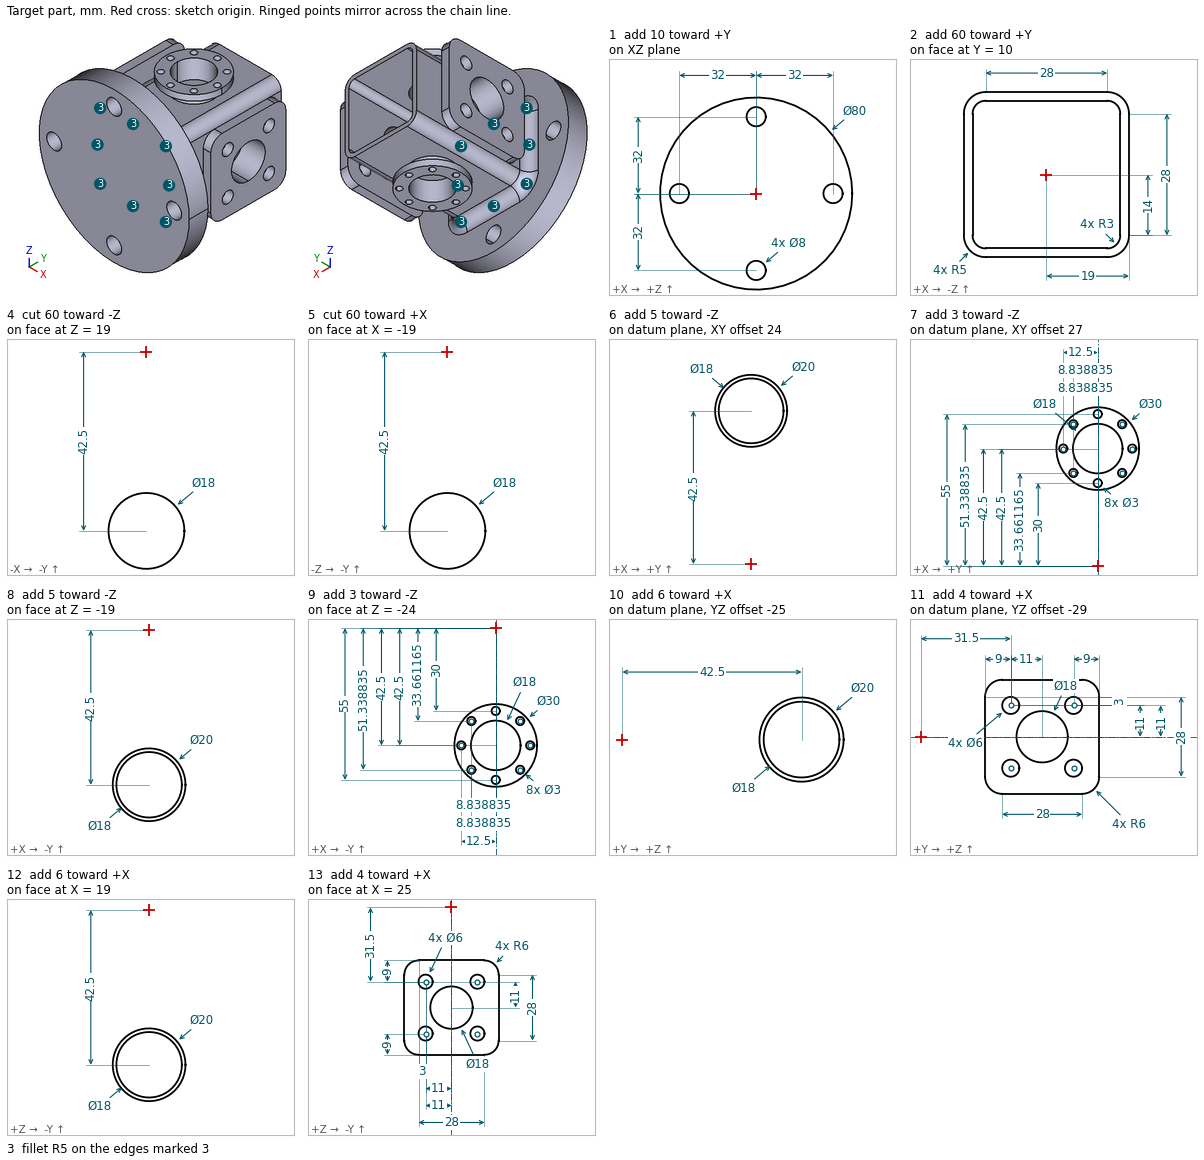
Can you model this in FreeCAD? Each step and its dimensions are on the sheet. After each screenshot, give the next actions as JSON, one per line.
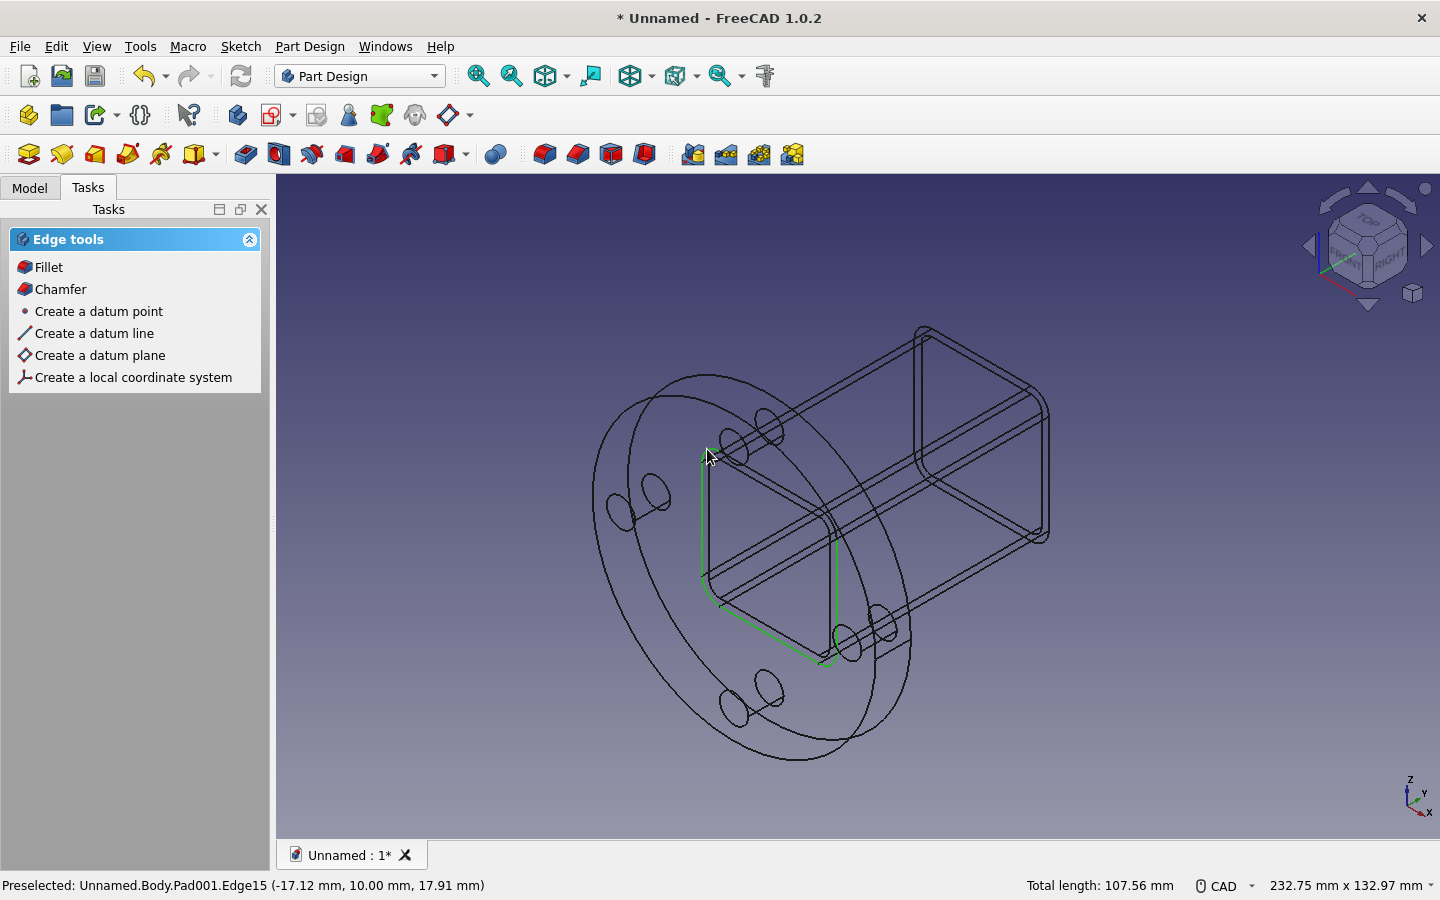
{"action": "left_click", "coordinate": [769, 479], "text": "ctrl"}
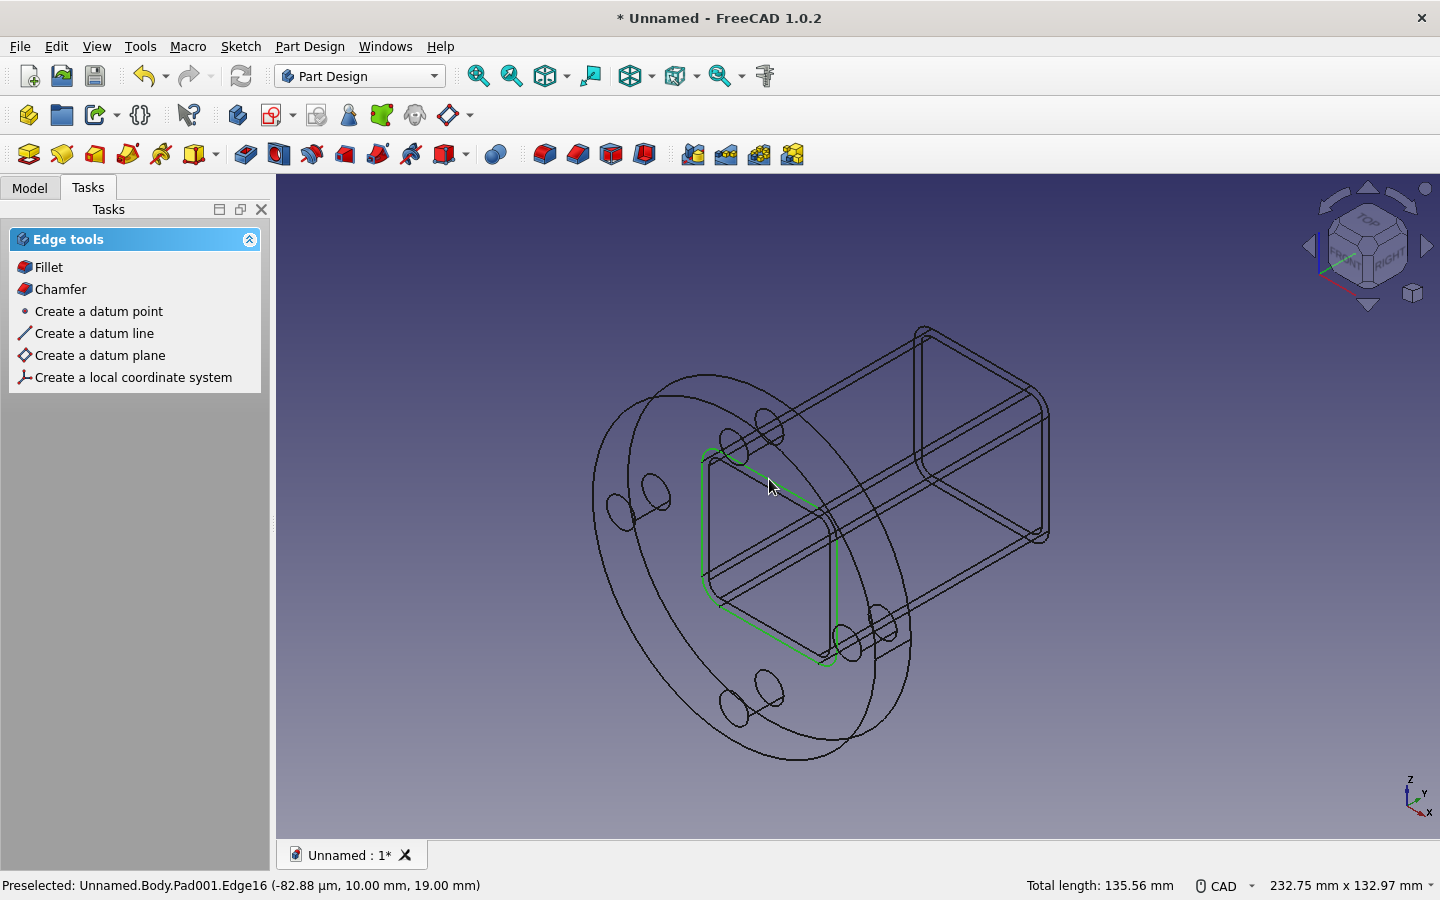
{"action": "key", "text": "2"}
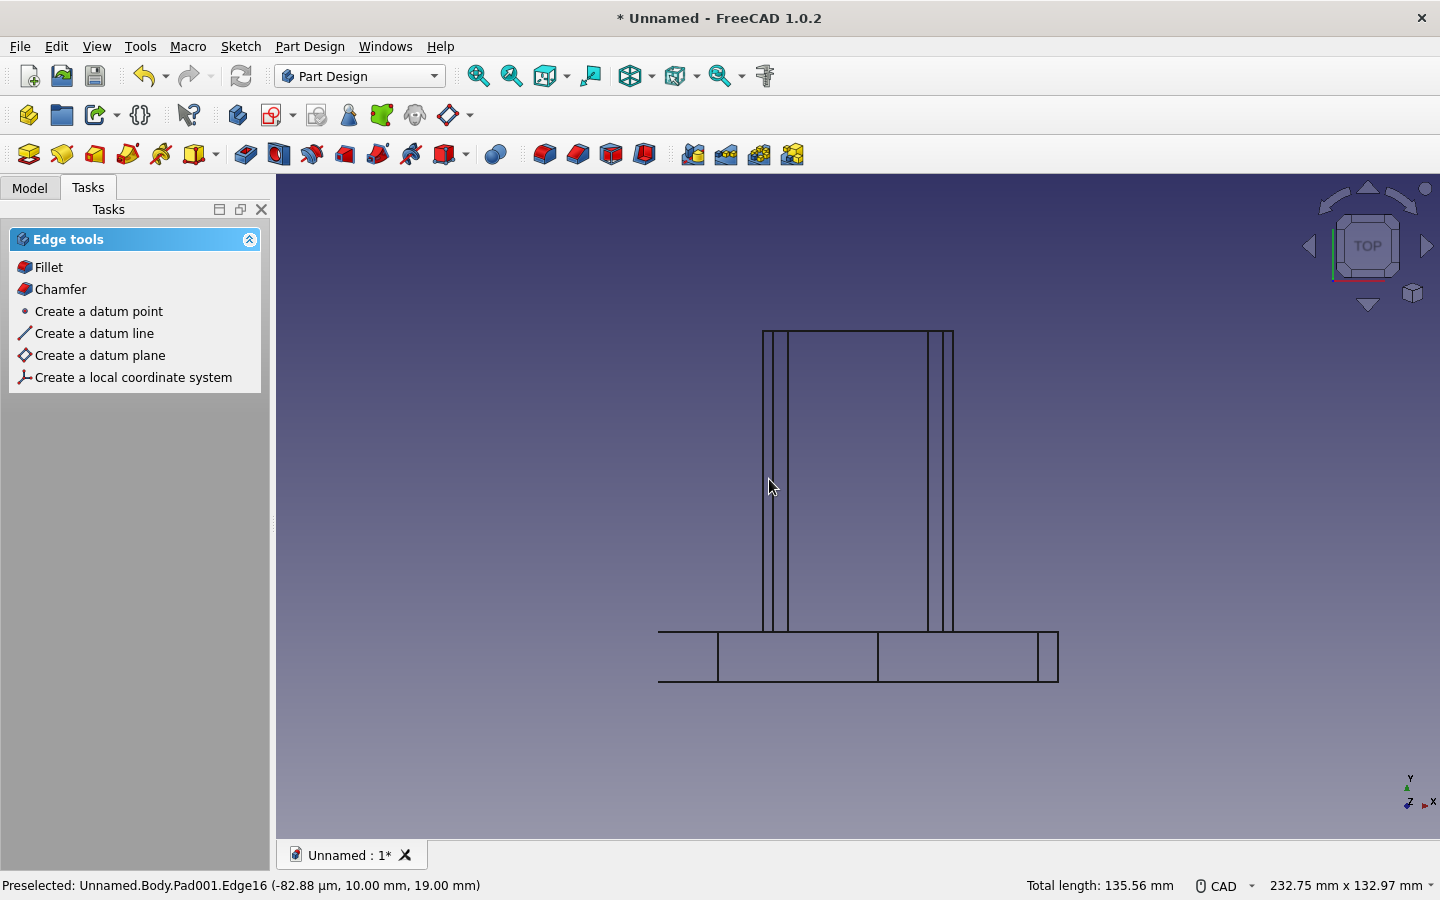
{"action": "key", "text": "1"}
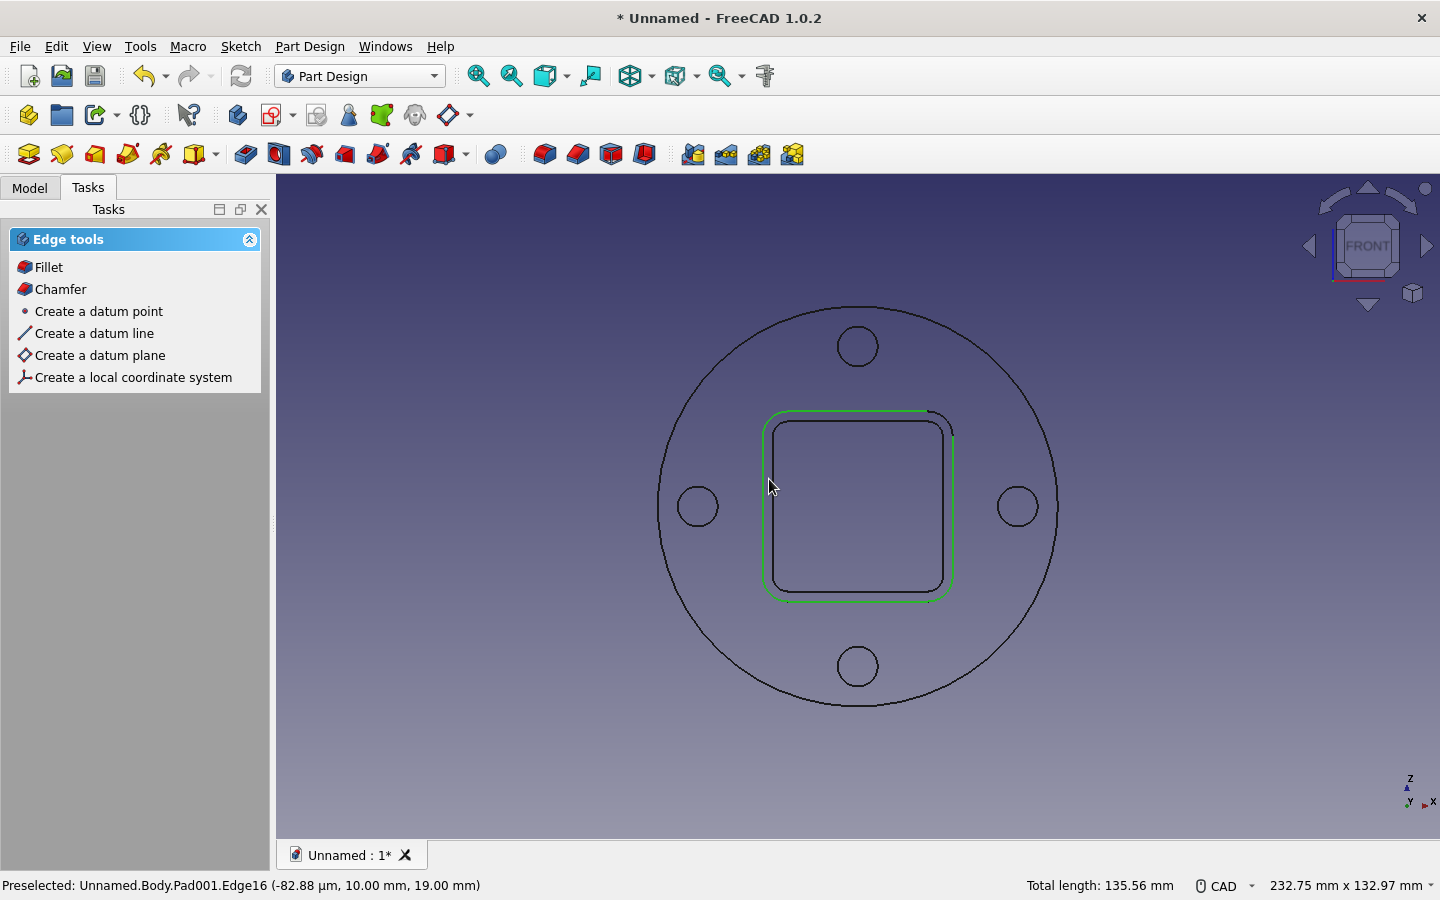
{"action": "left_click", "coordinate": [946, 418], "text": "ctrl"}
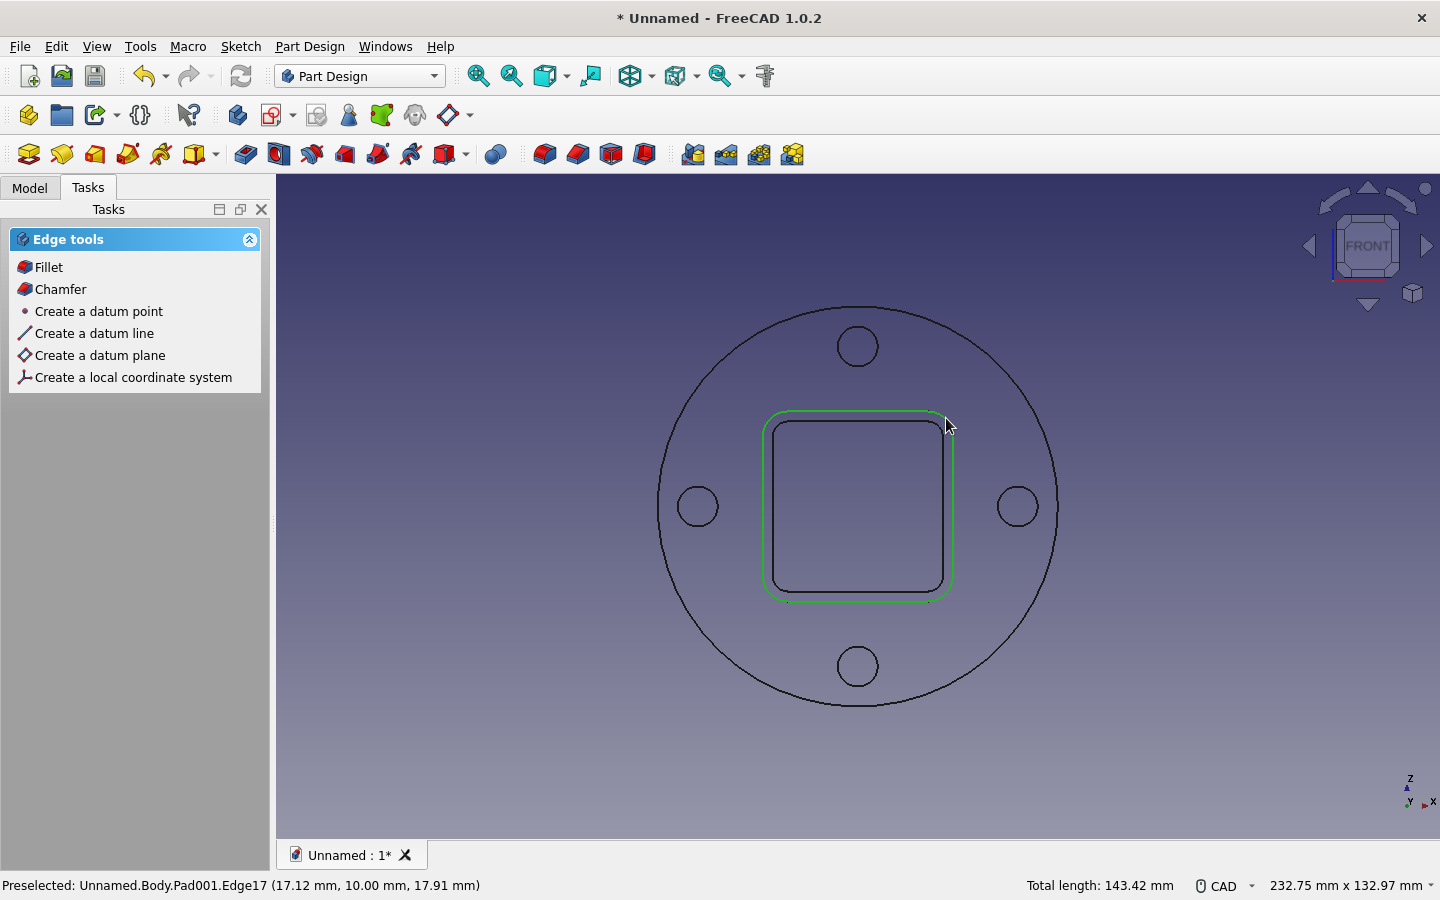
{"action": "key", "text": "v 1"}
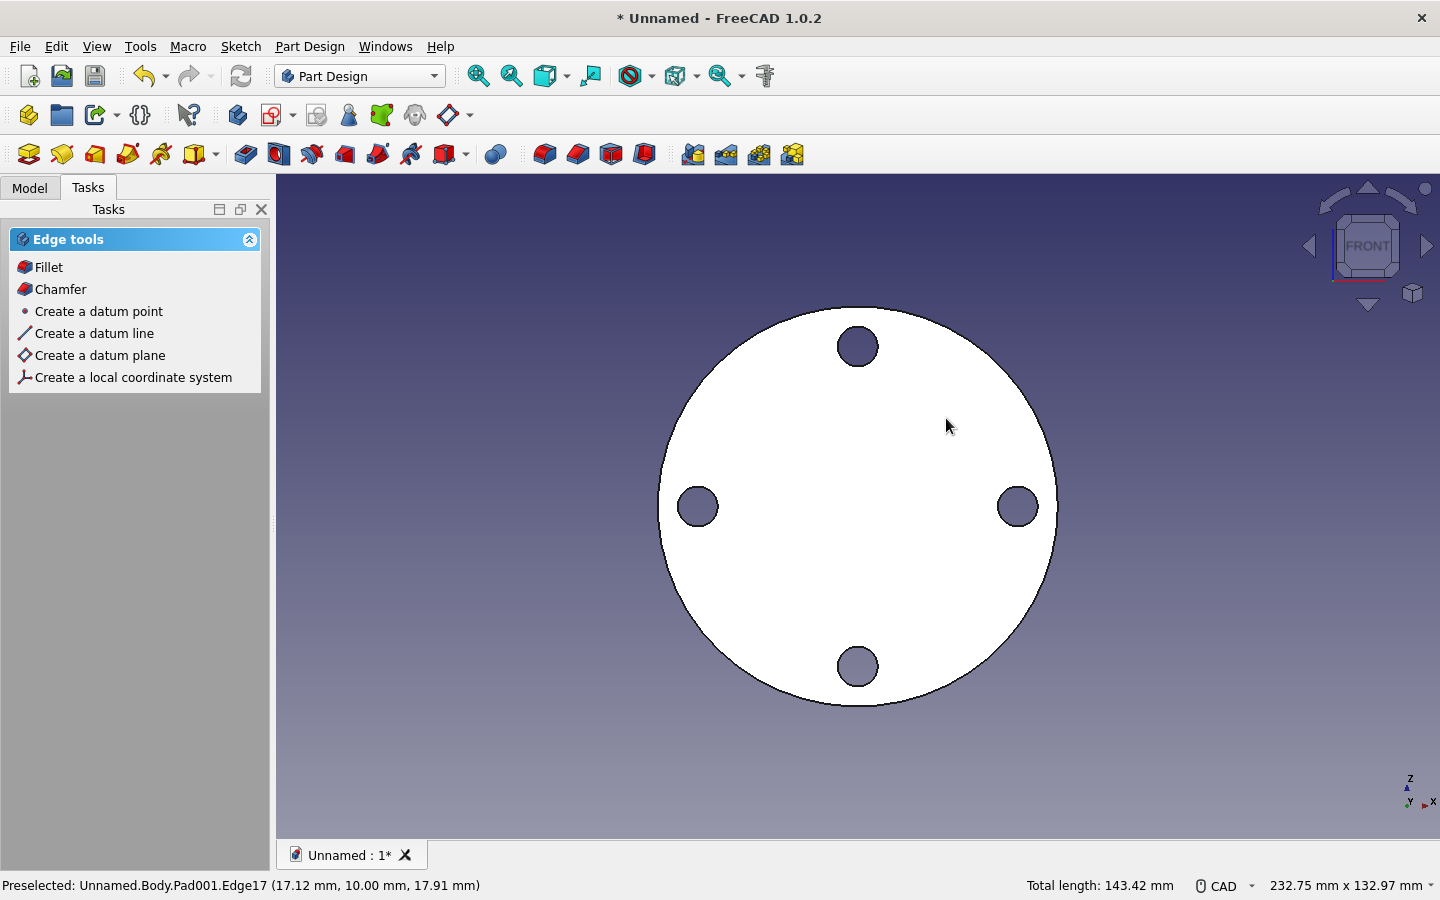
{"action": "left_click", "coordinate": [545, 154]}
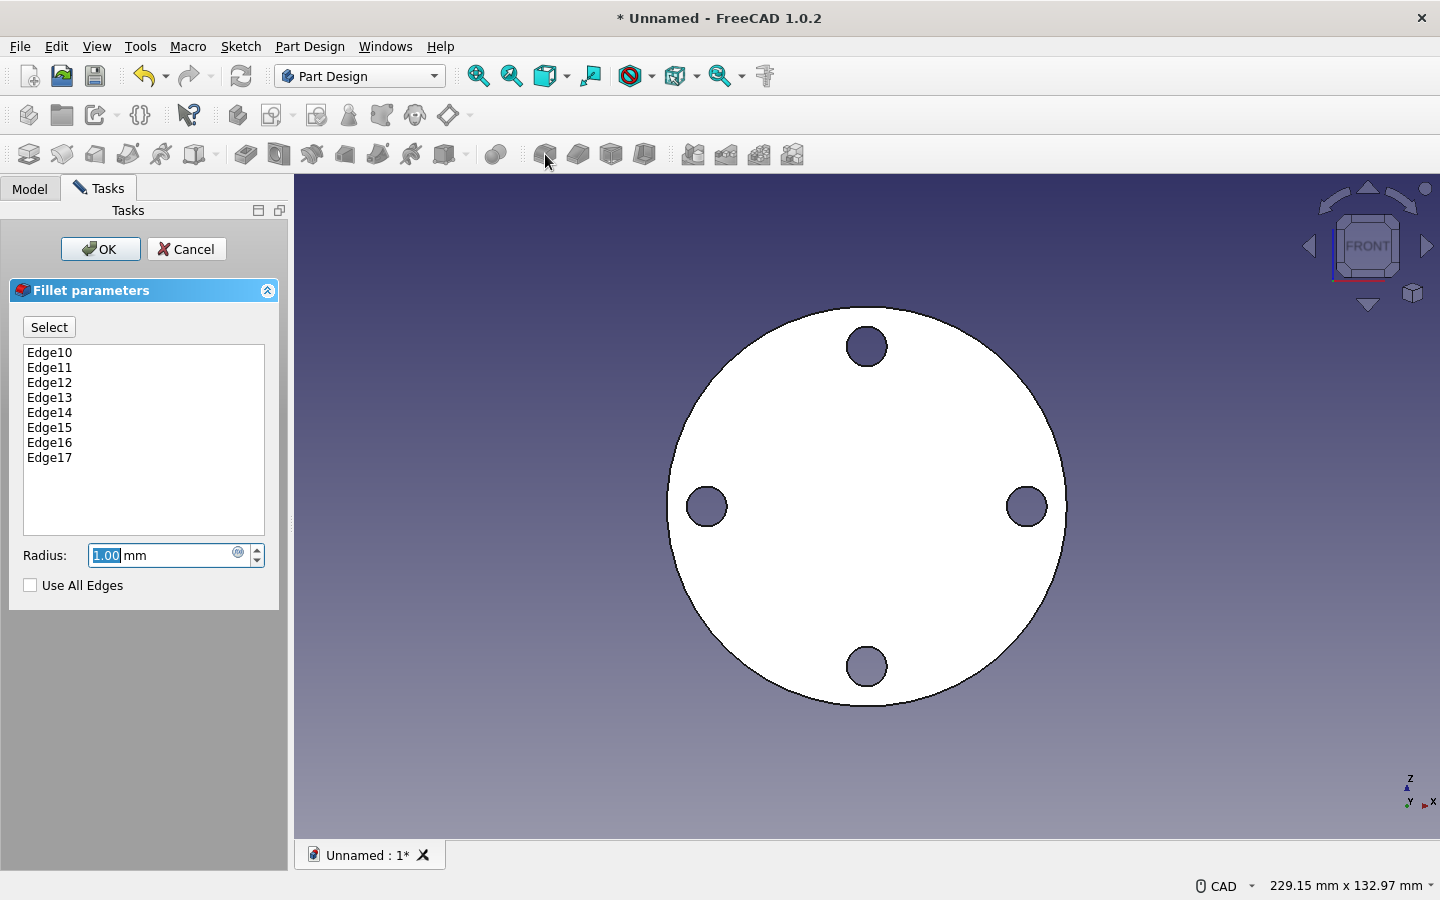
{"action": "type", "text": "5"}
{"action": "key", "text": "Tab"}